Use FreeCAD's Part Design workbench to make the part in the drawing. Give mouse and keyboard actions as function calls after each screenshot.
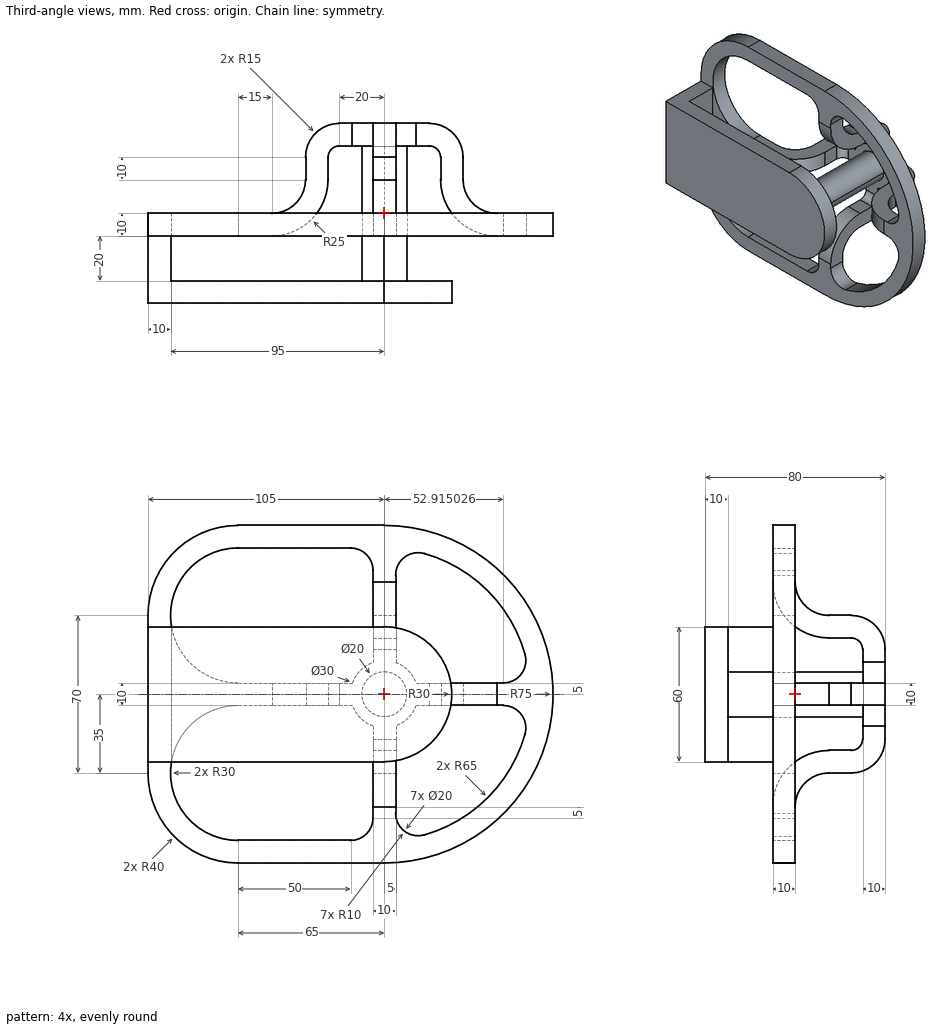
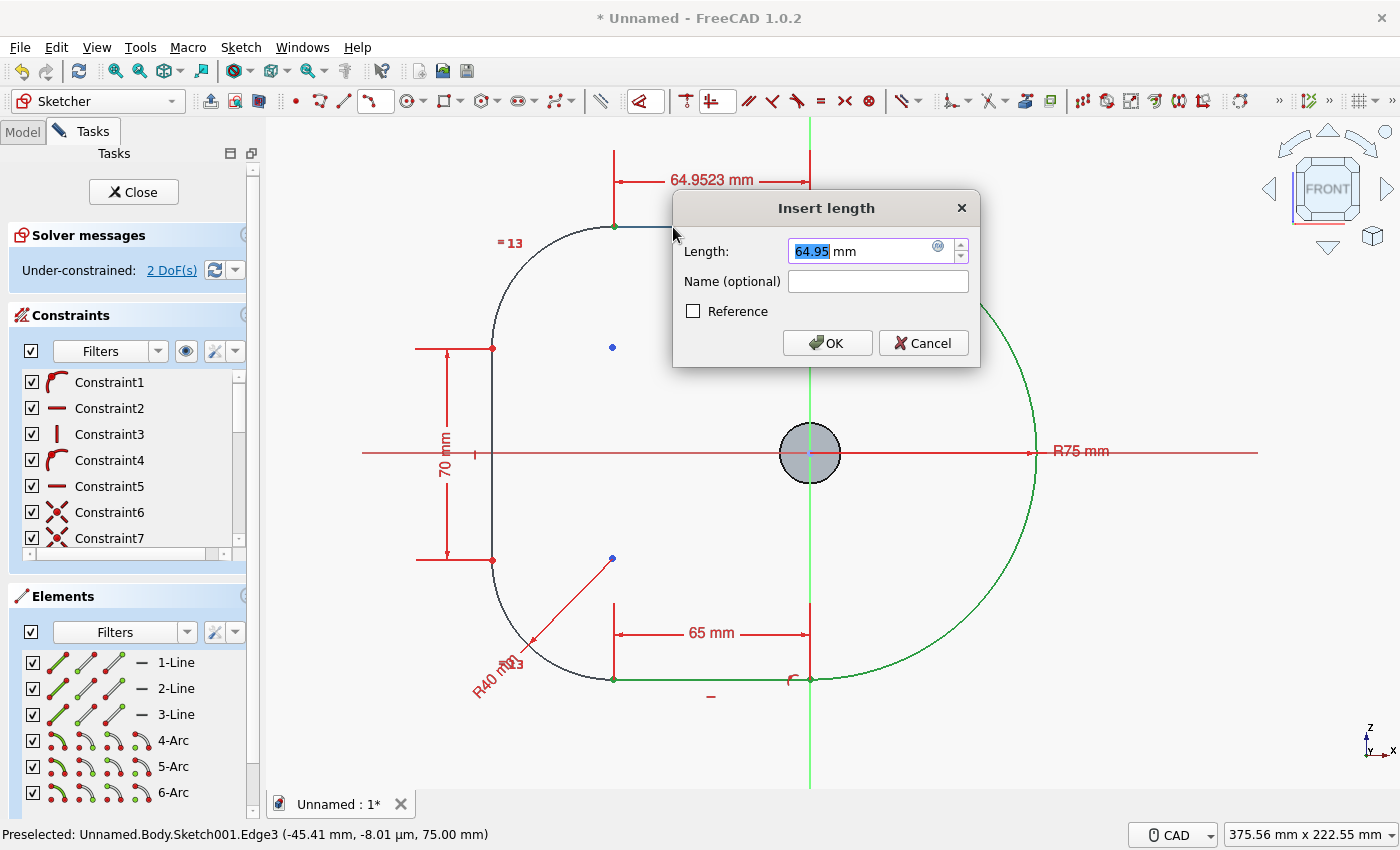
text(65)
key(Return)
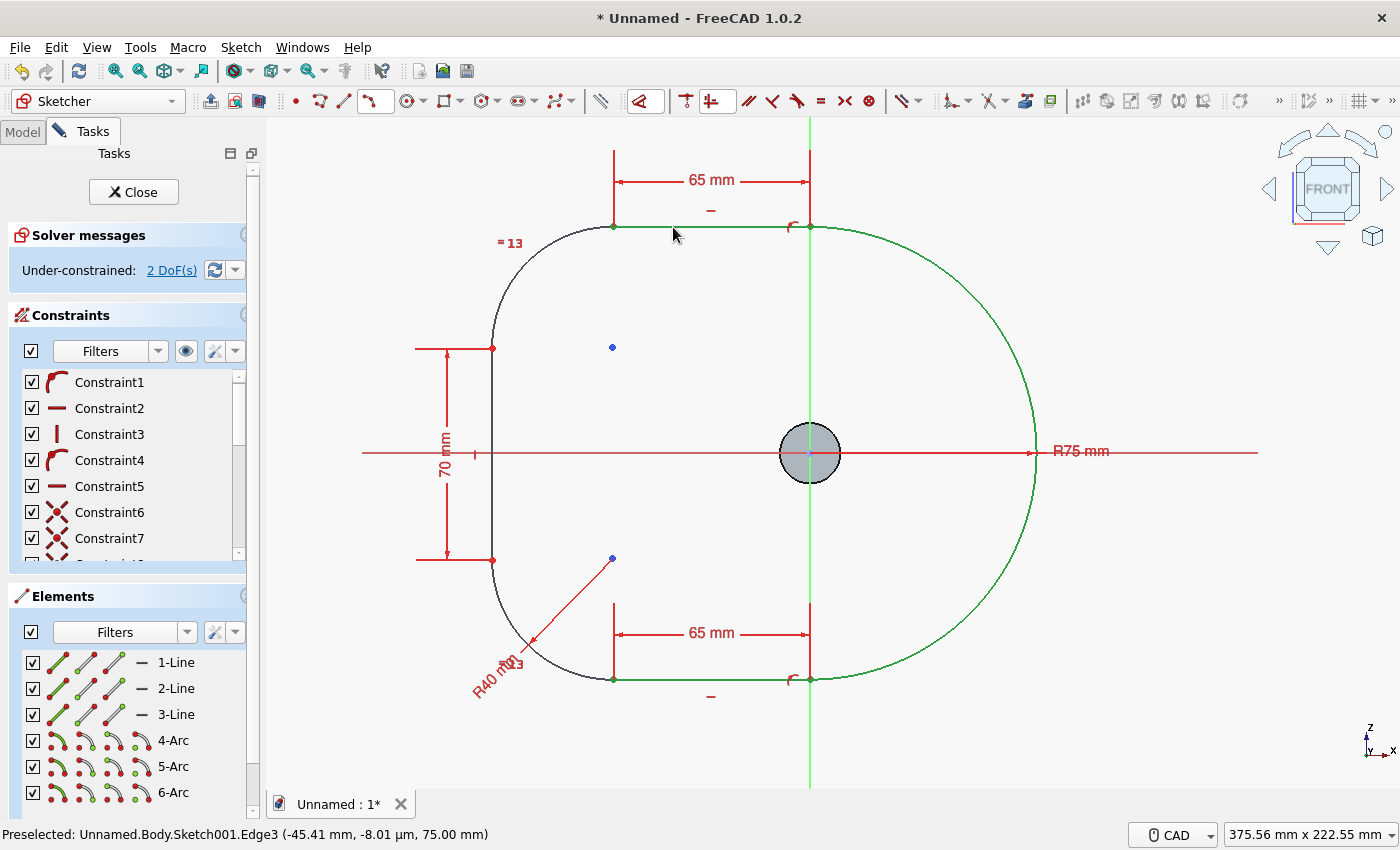
click(492, 560)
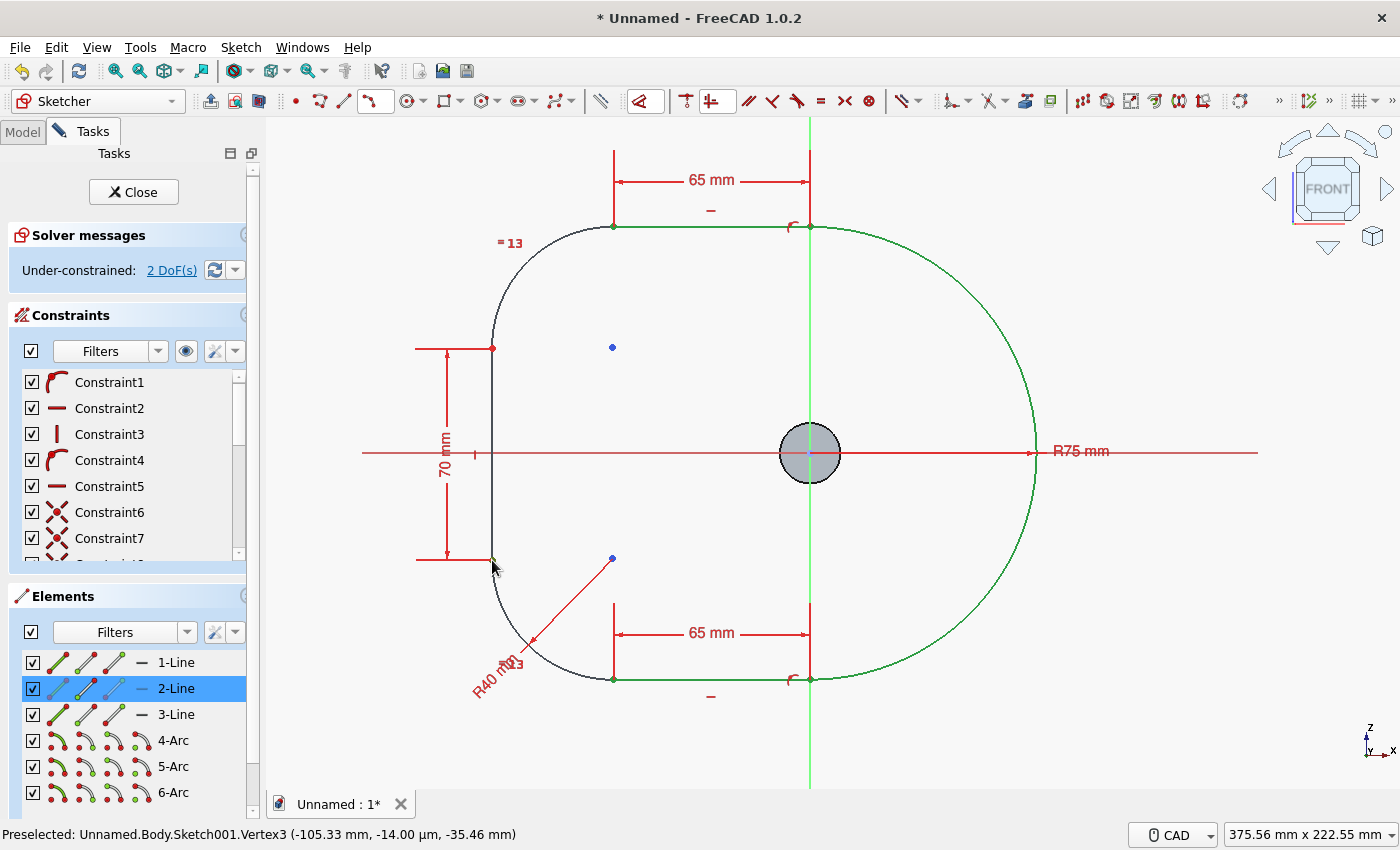
click(658, 102)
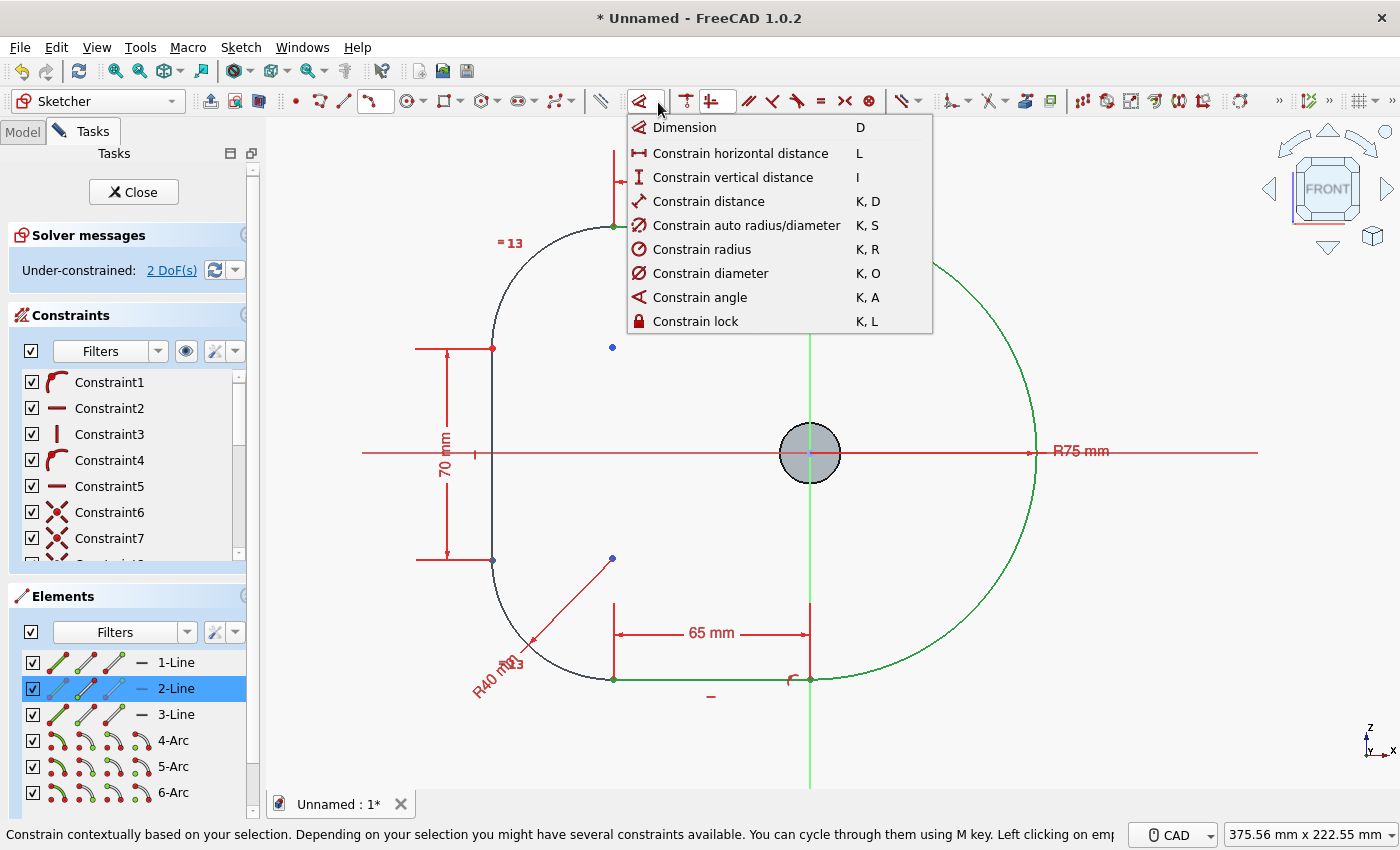
click(780, 177)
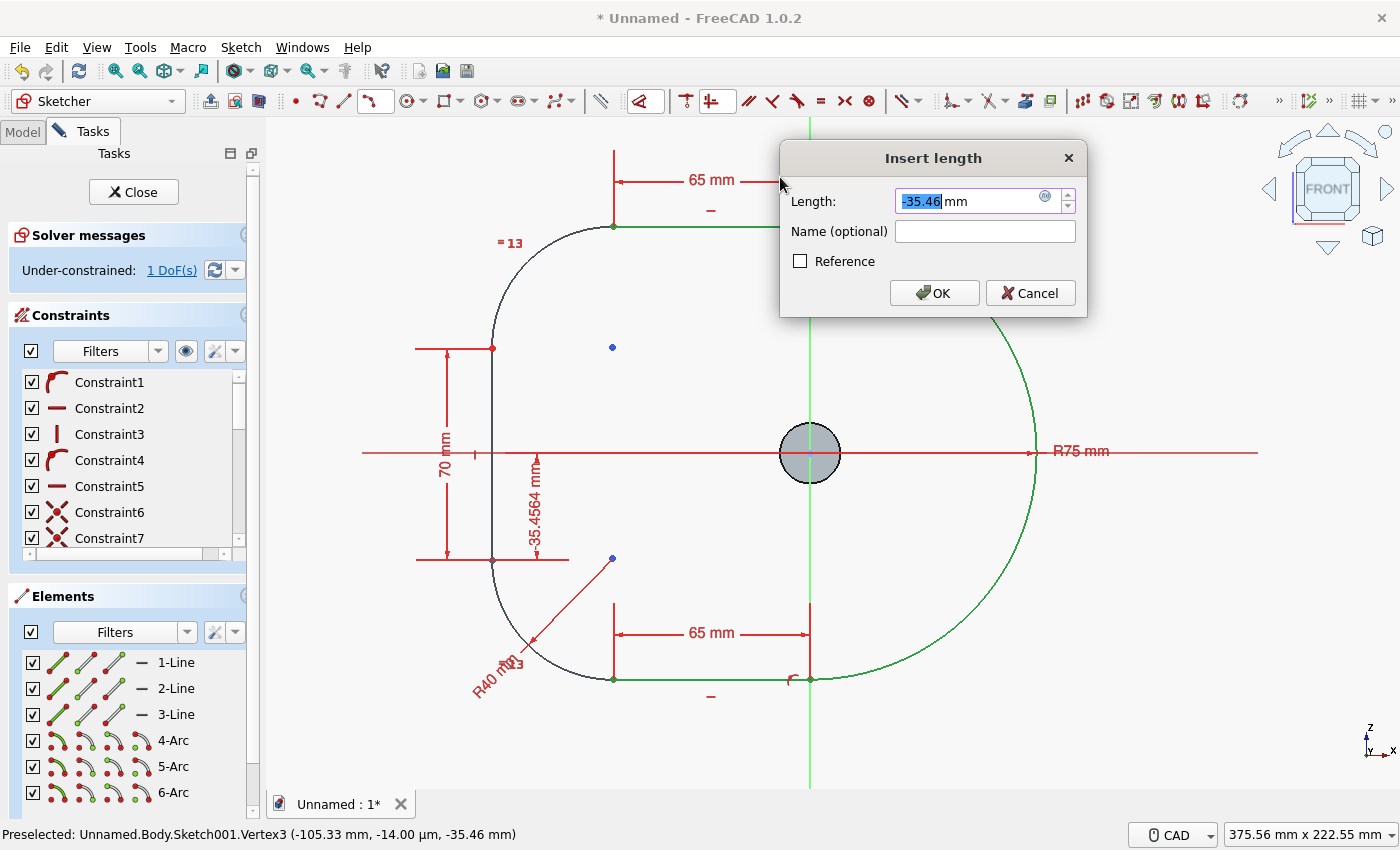
text(-35)
key(Return)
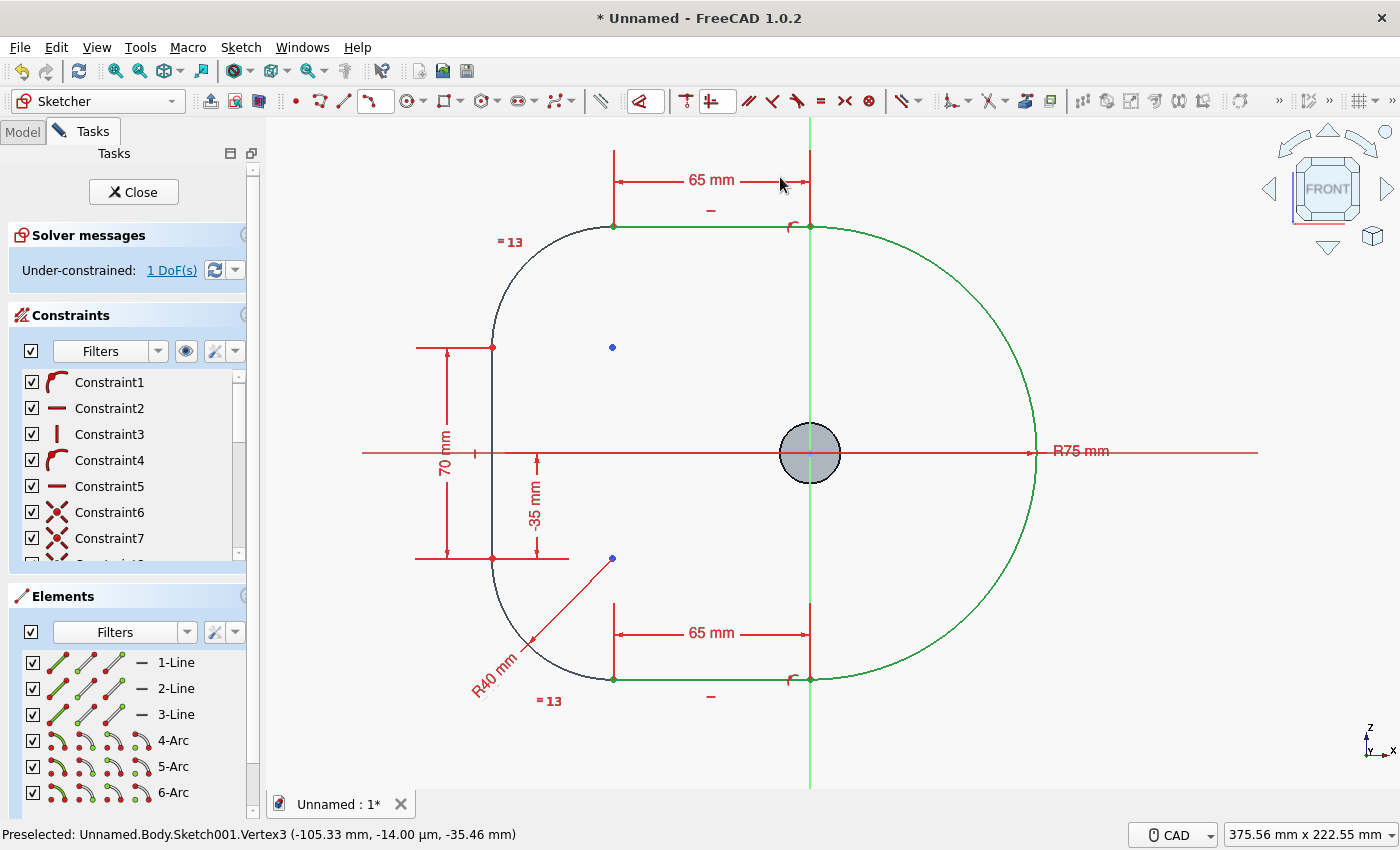
click(613, 559)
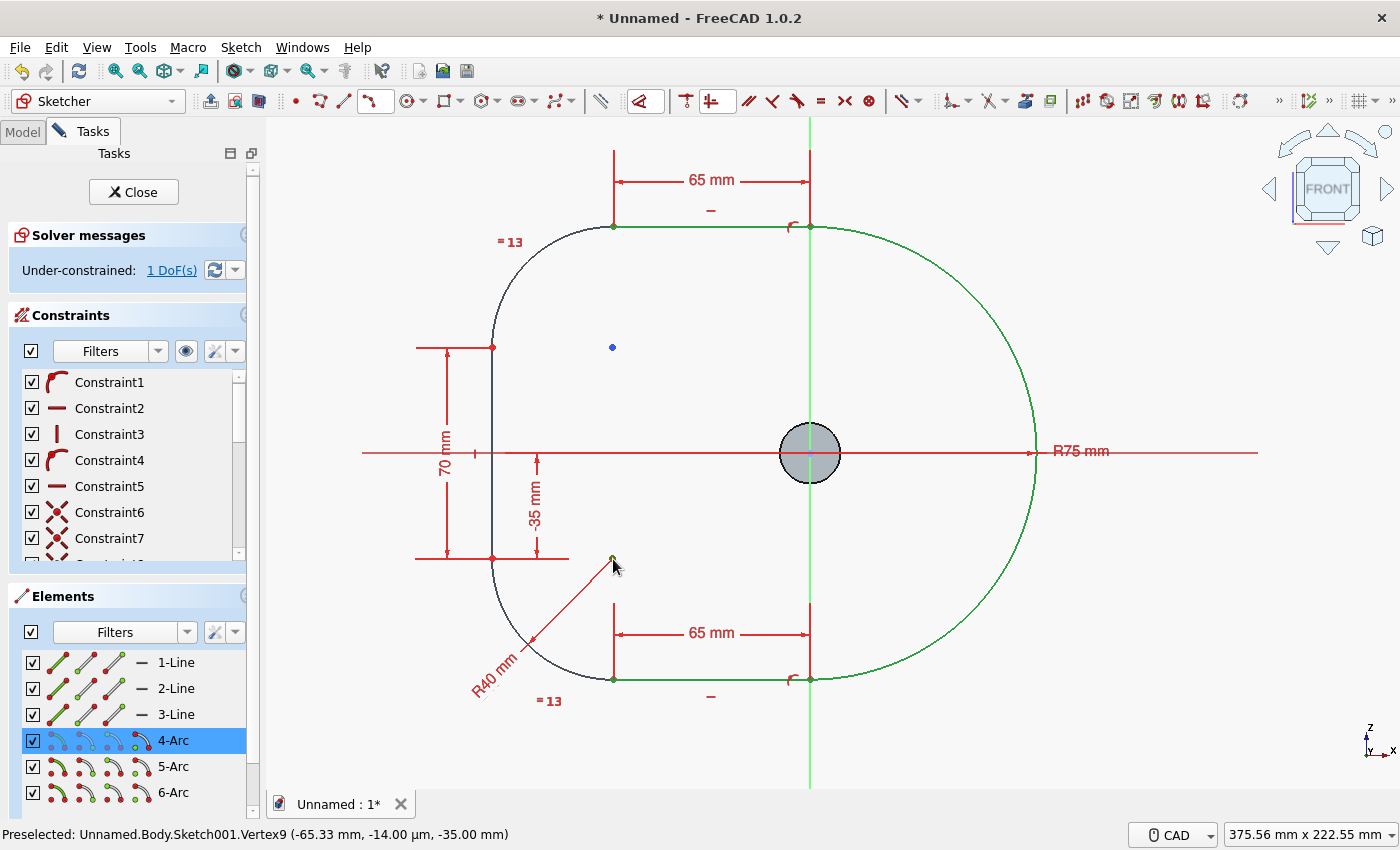
click(658, 102)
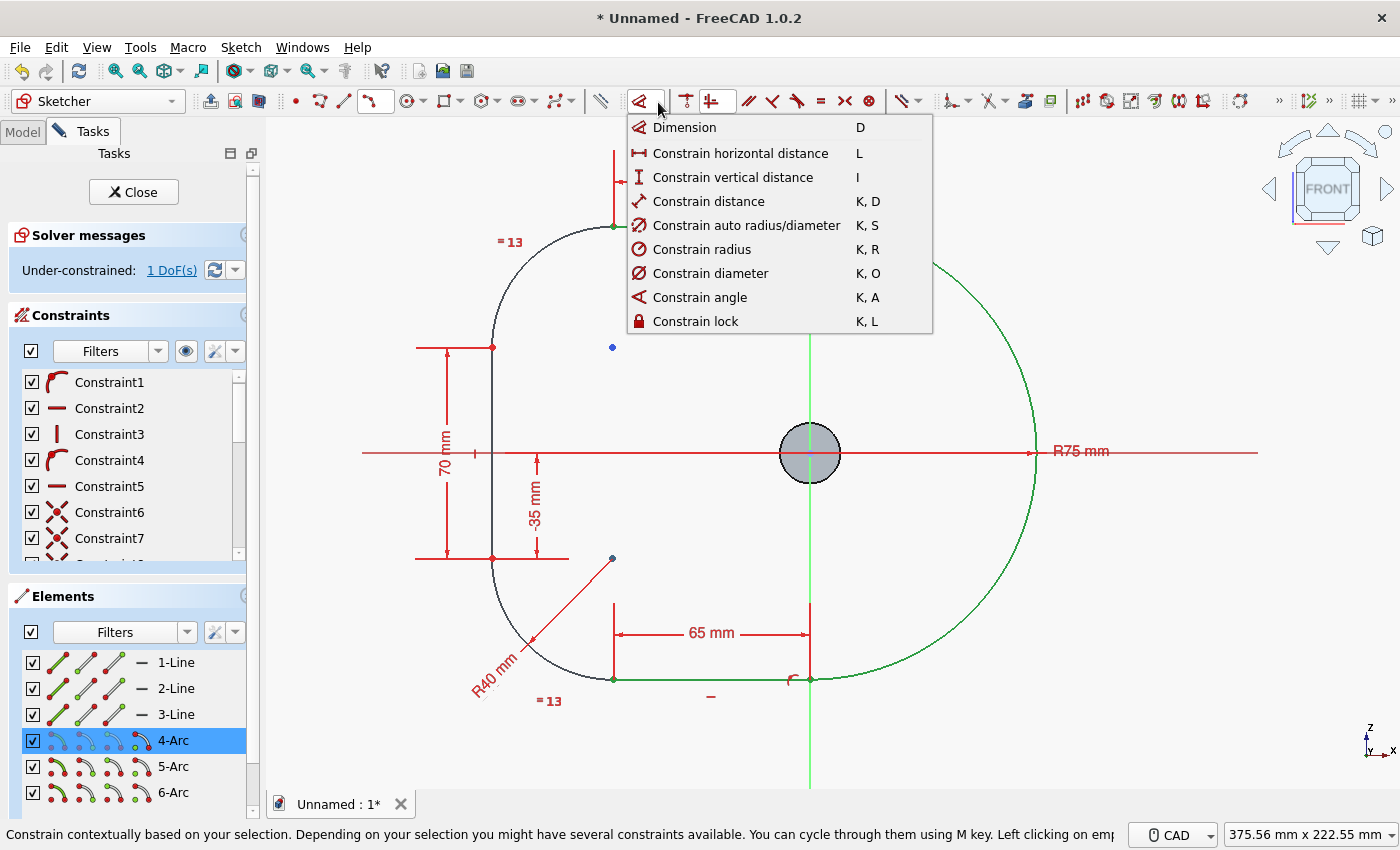
click(780, 153)